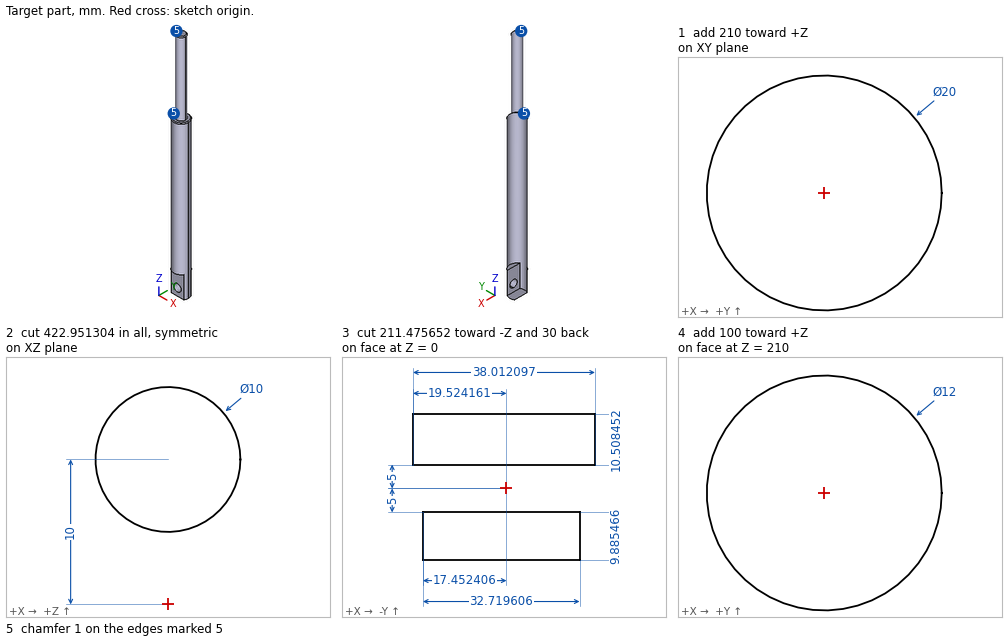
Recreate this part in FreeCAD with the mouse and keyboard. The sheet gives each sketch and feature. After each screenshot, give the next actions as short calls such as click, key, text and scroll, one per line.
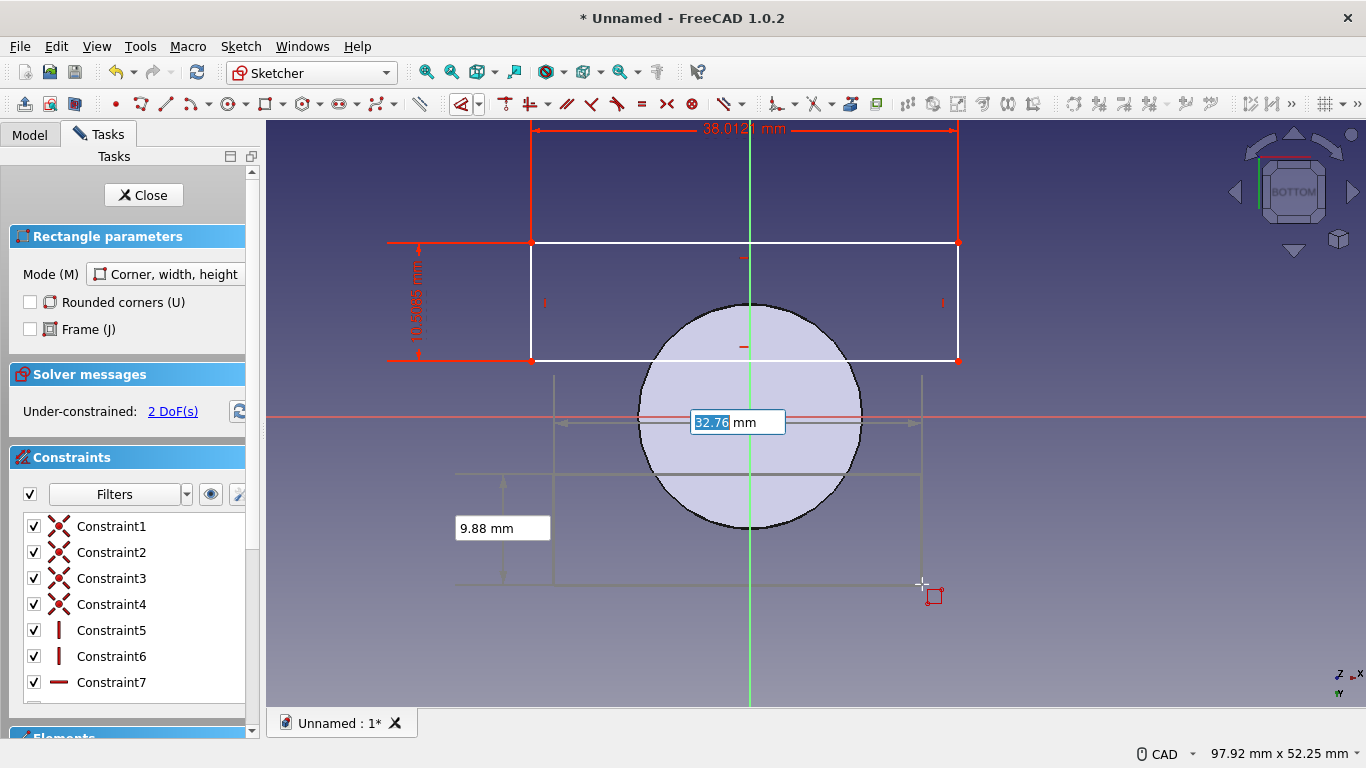
text(32.719606)
key(Tab)
text(9.885466)
key(Return)
key(Escape)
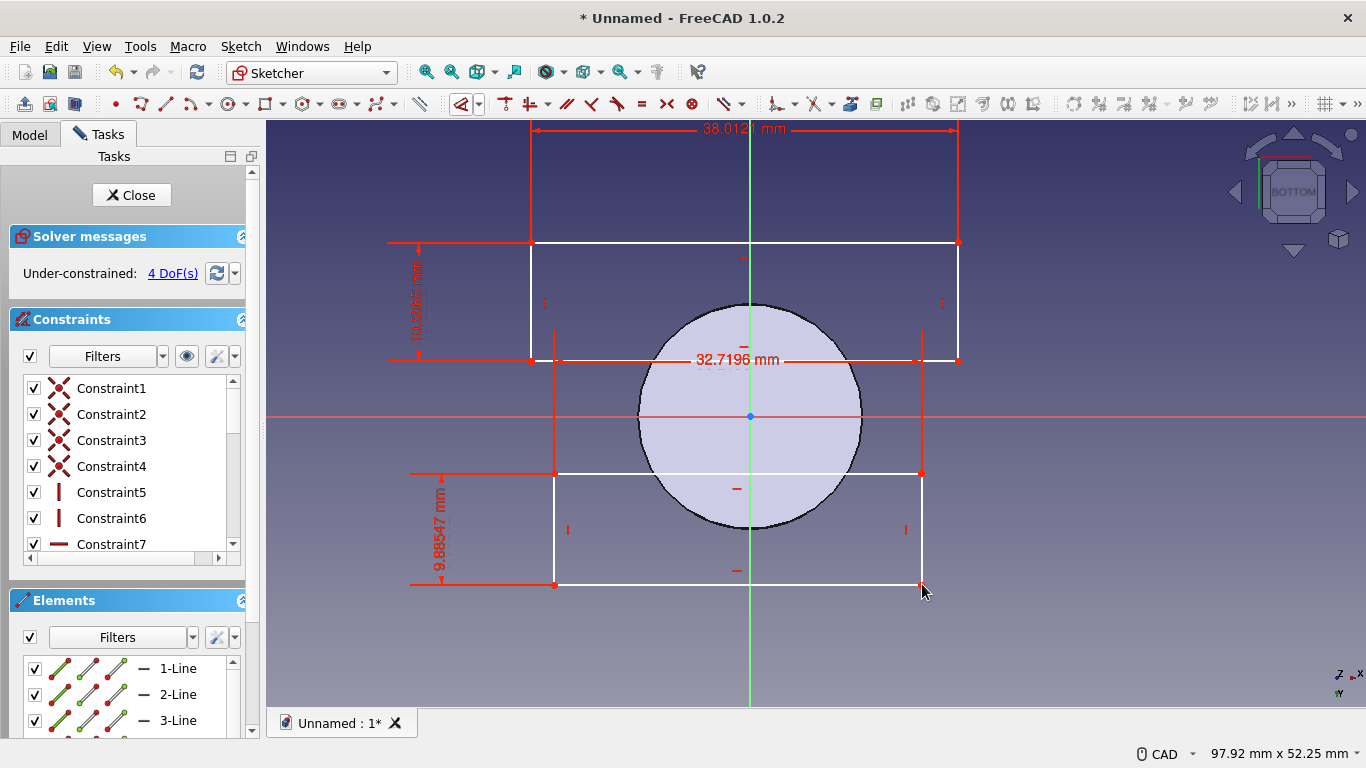
click(531, 361)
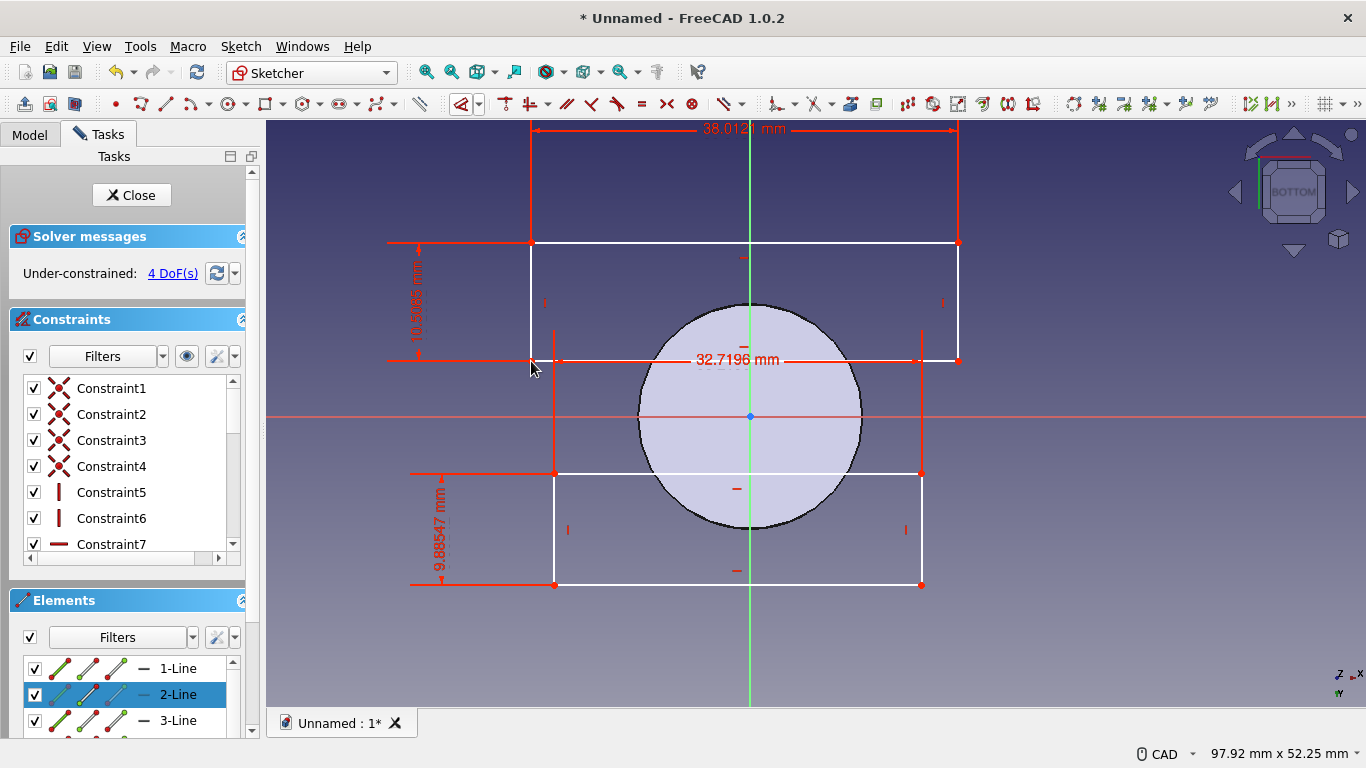
key(i)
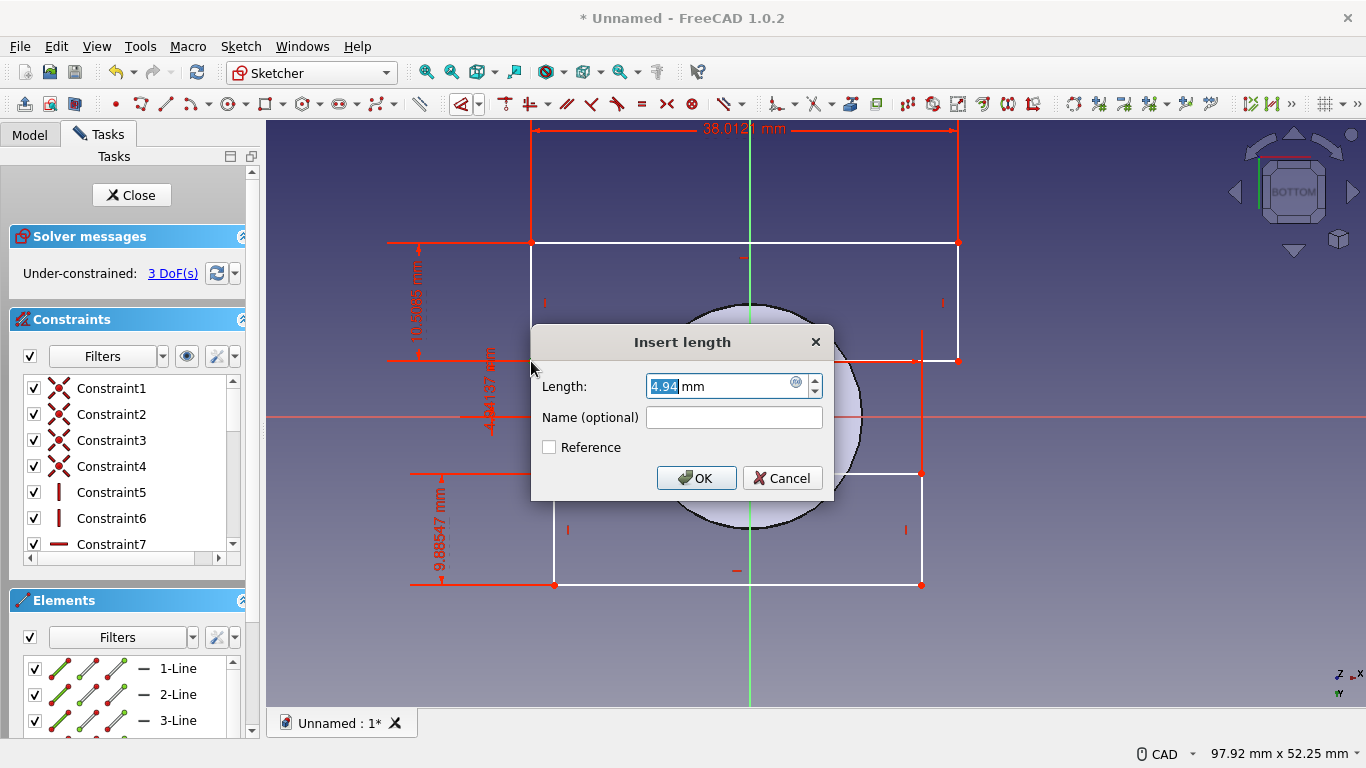
text(5)
key(Return)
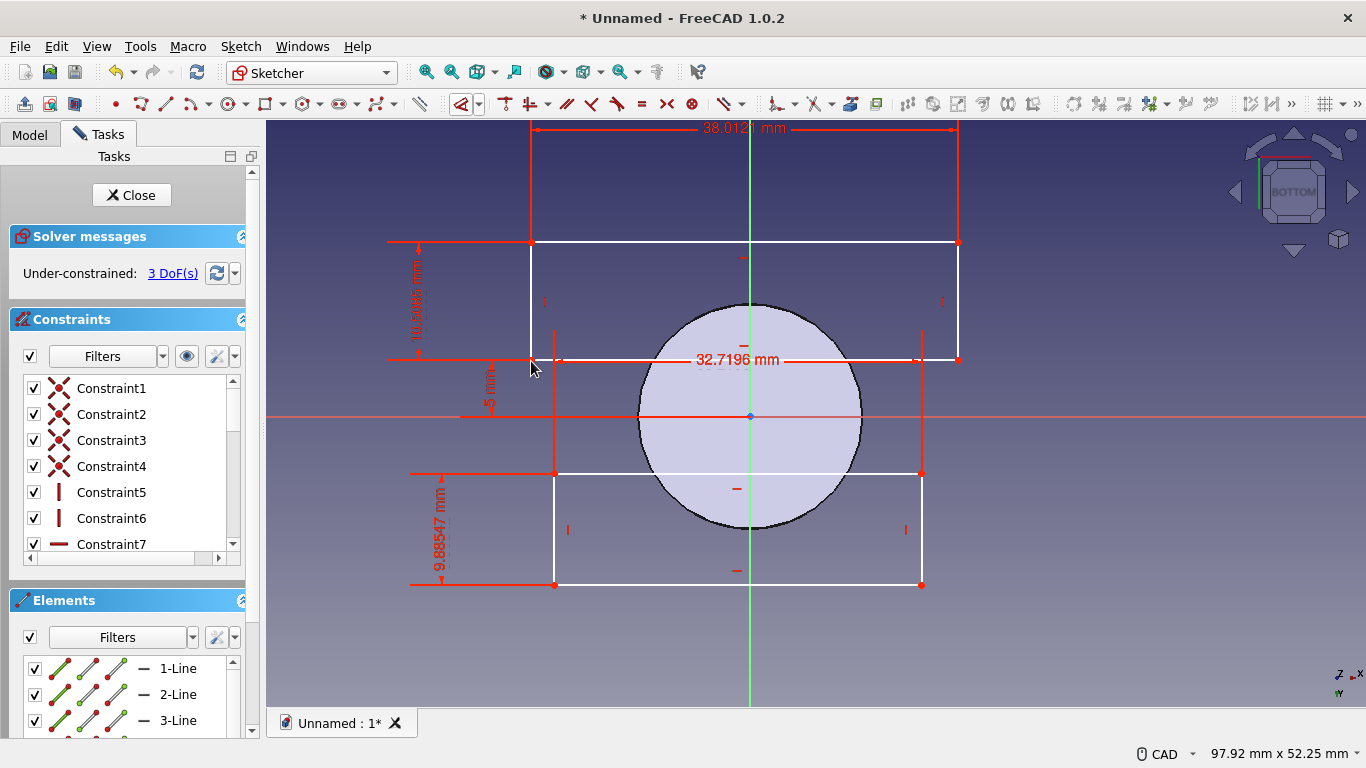
click(554, 474)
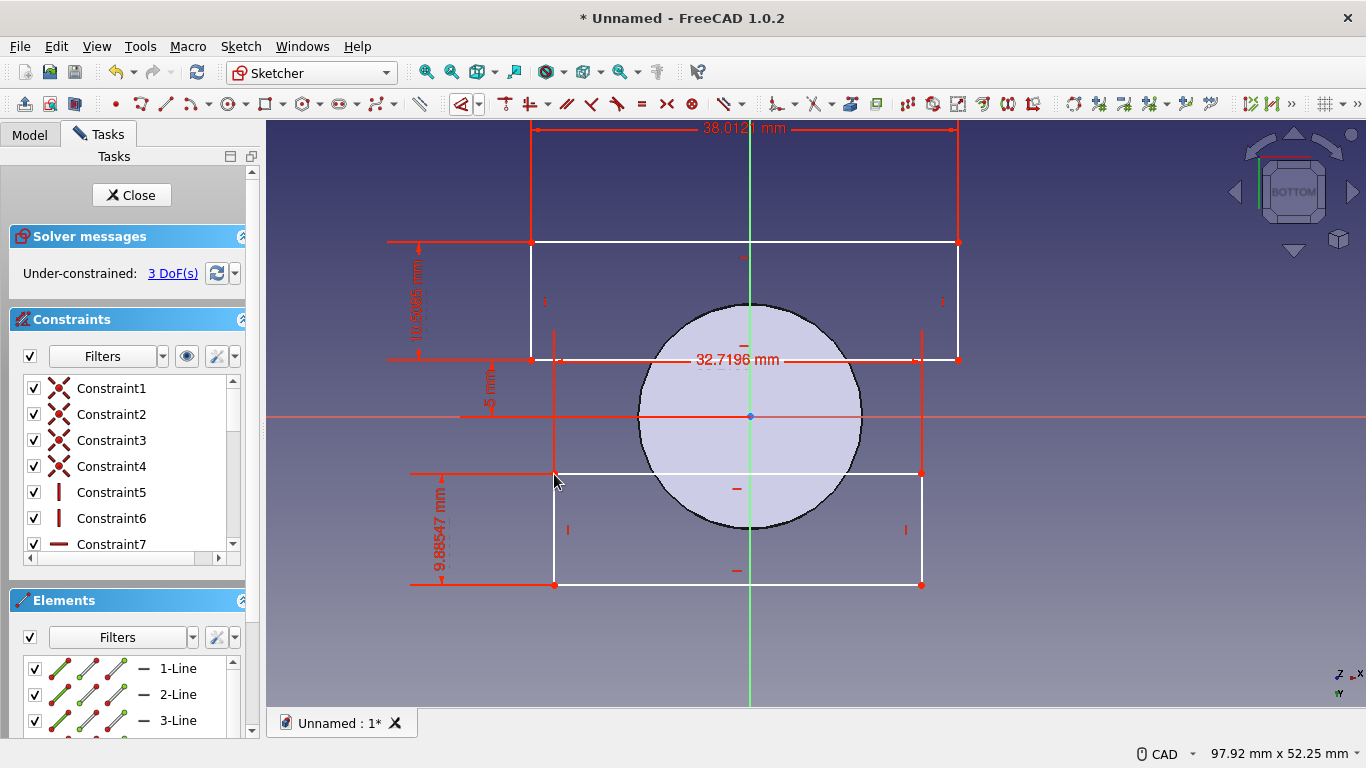
click(478, 104)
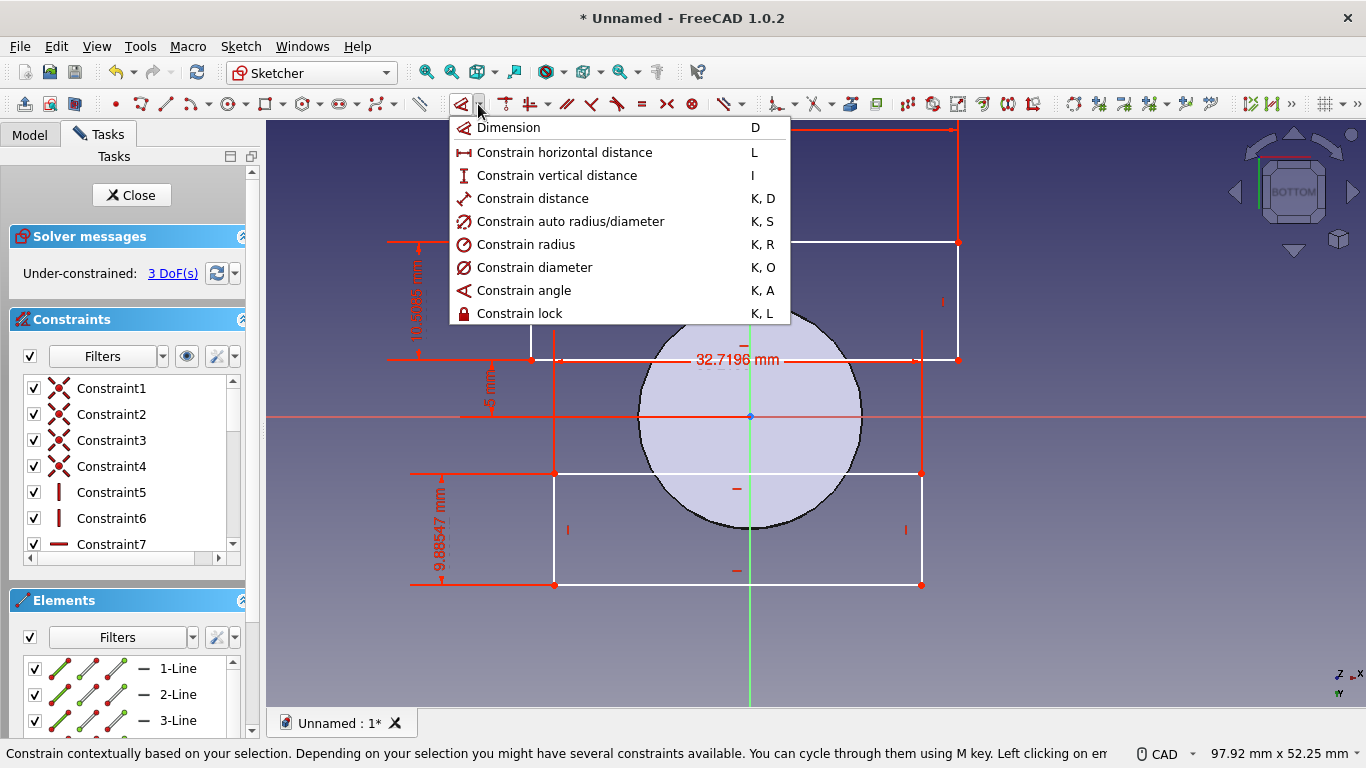
click(620, 176)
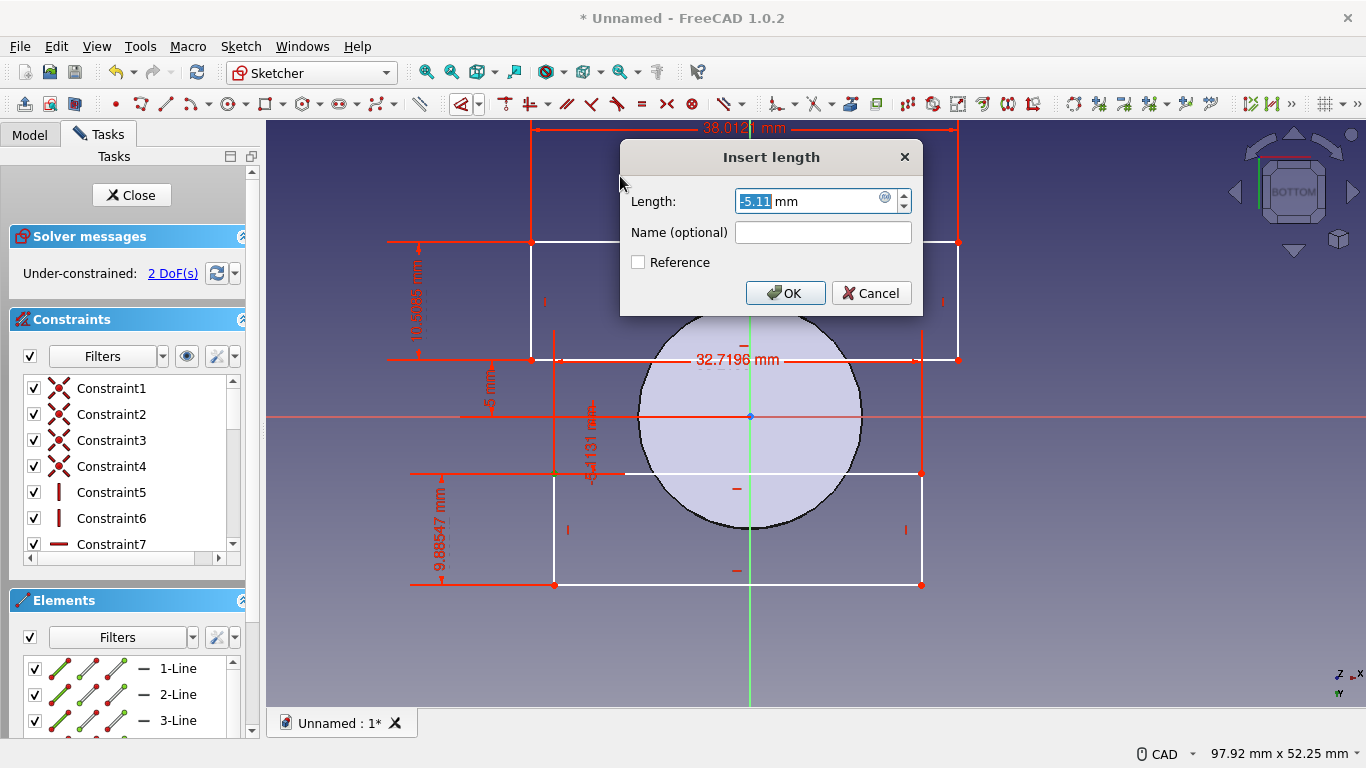
text(-5)
key(Return)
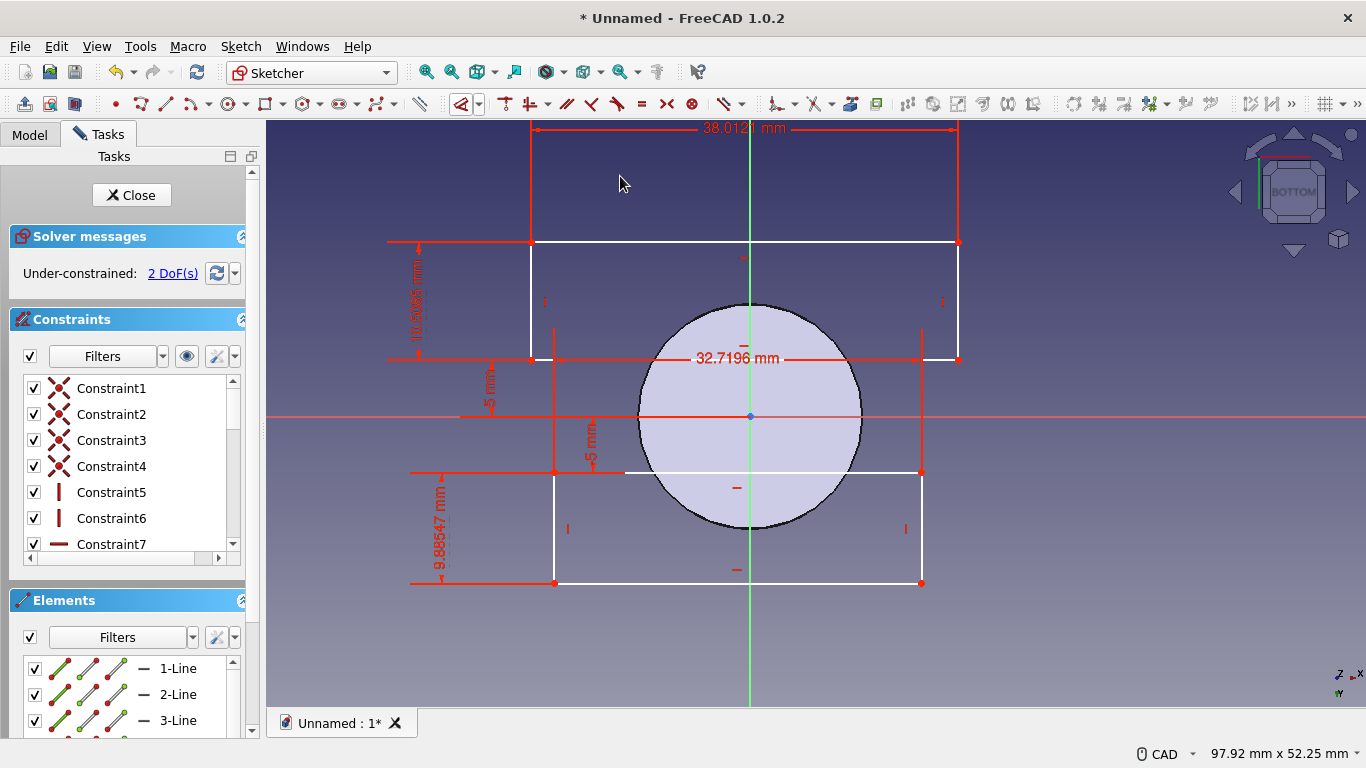
click(531, 242)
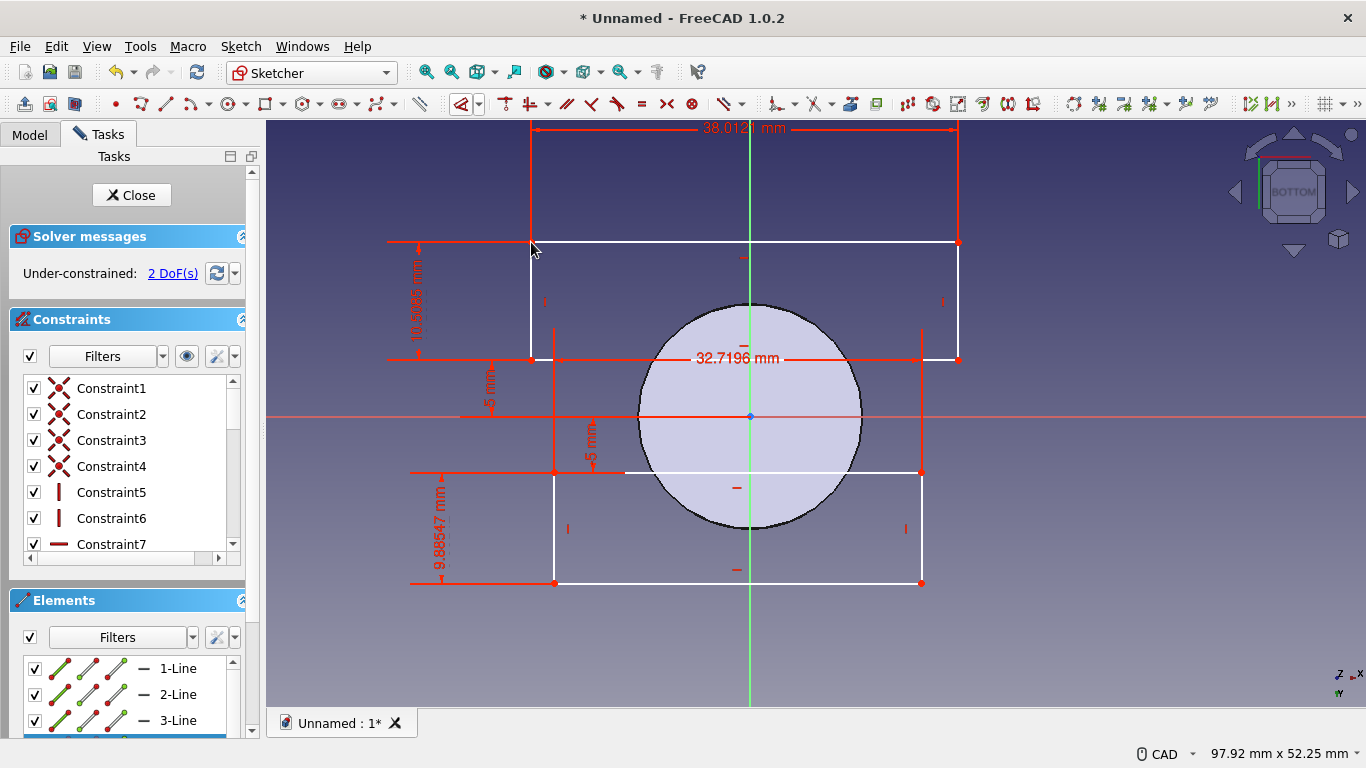
click(478, 104)